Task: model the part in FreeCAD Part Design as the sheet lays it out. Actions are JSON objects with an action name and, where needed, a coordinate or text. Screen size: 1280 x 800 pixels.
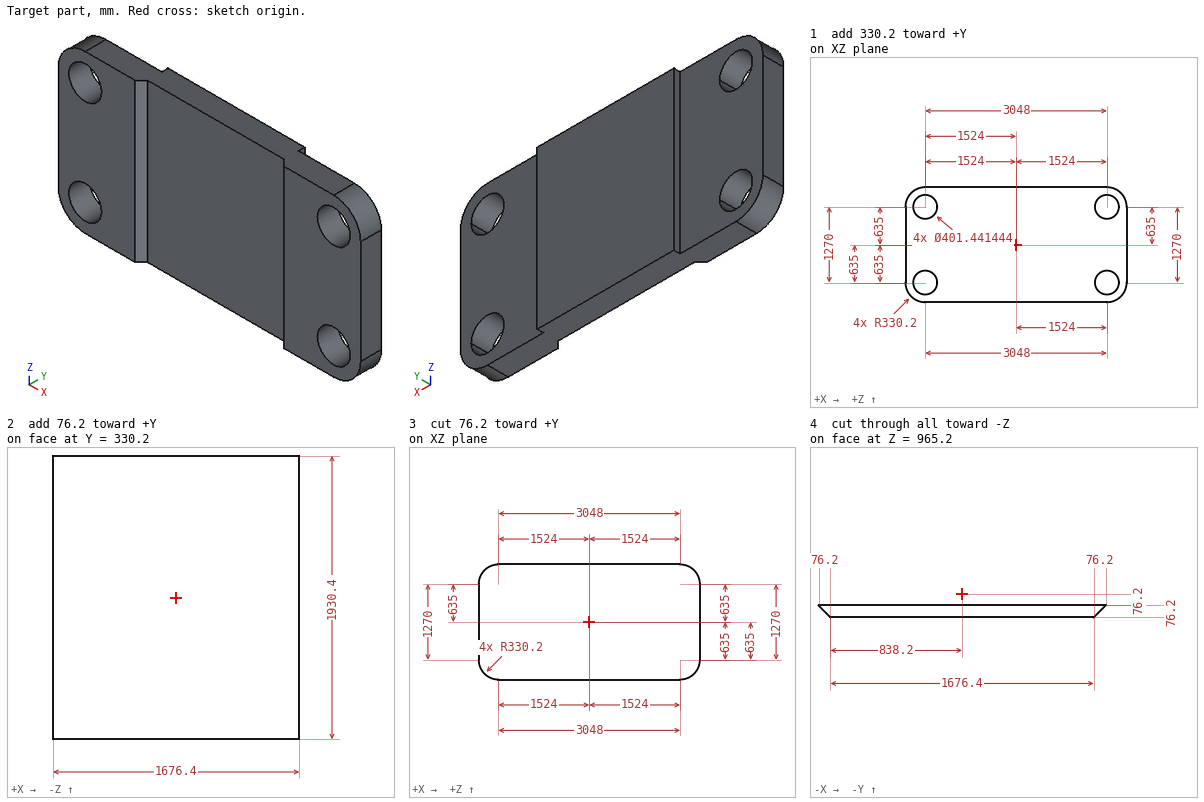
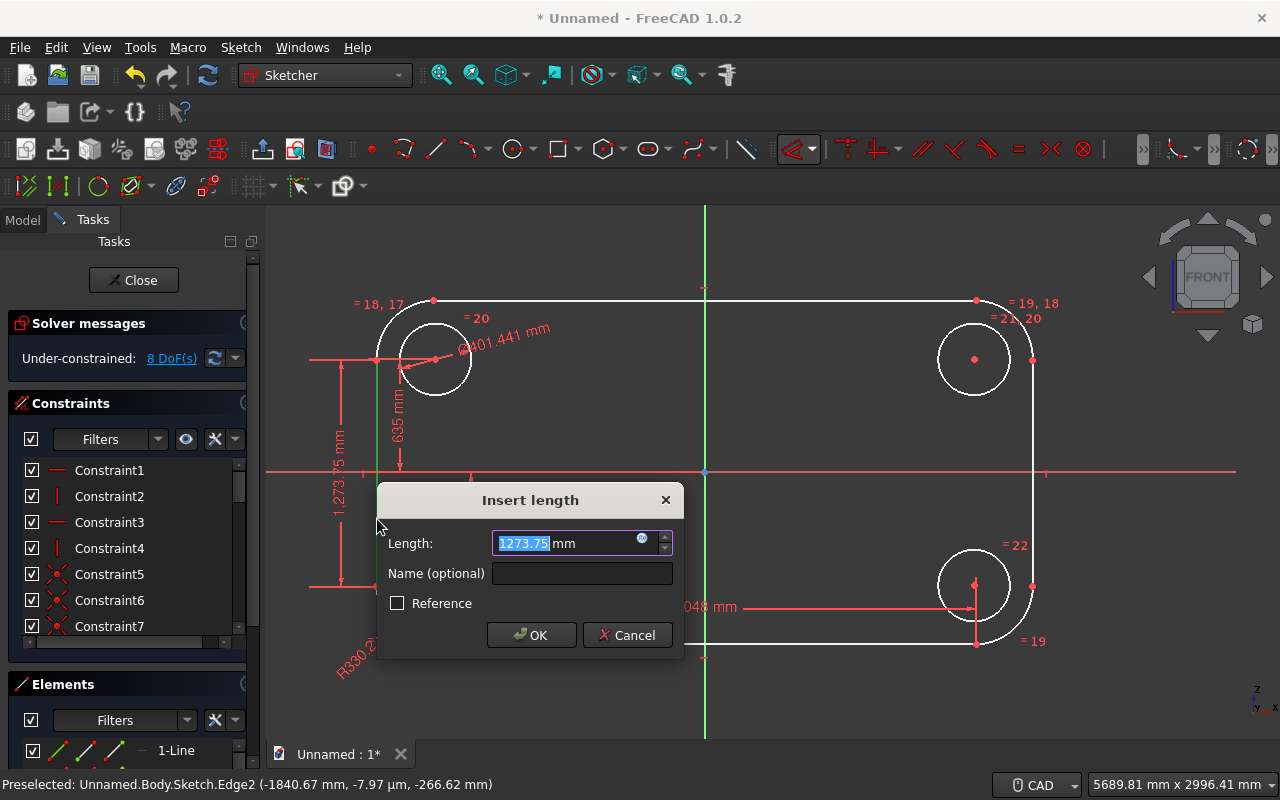
{"action": "type", "text": "1270"}
{"action": "key", "text": "Return"}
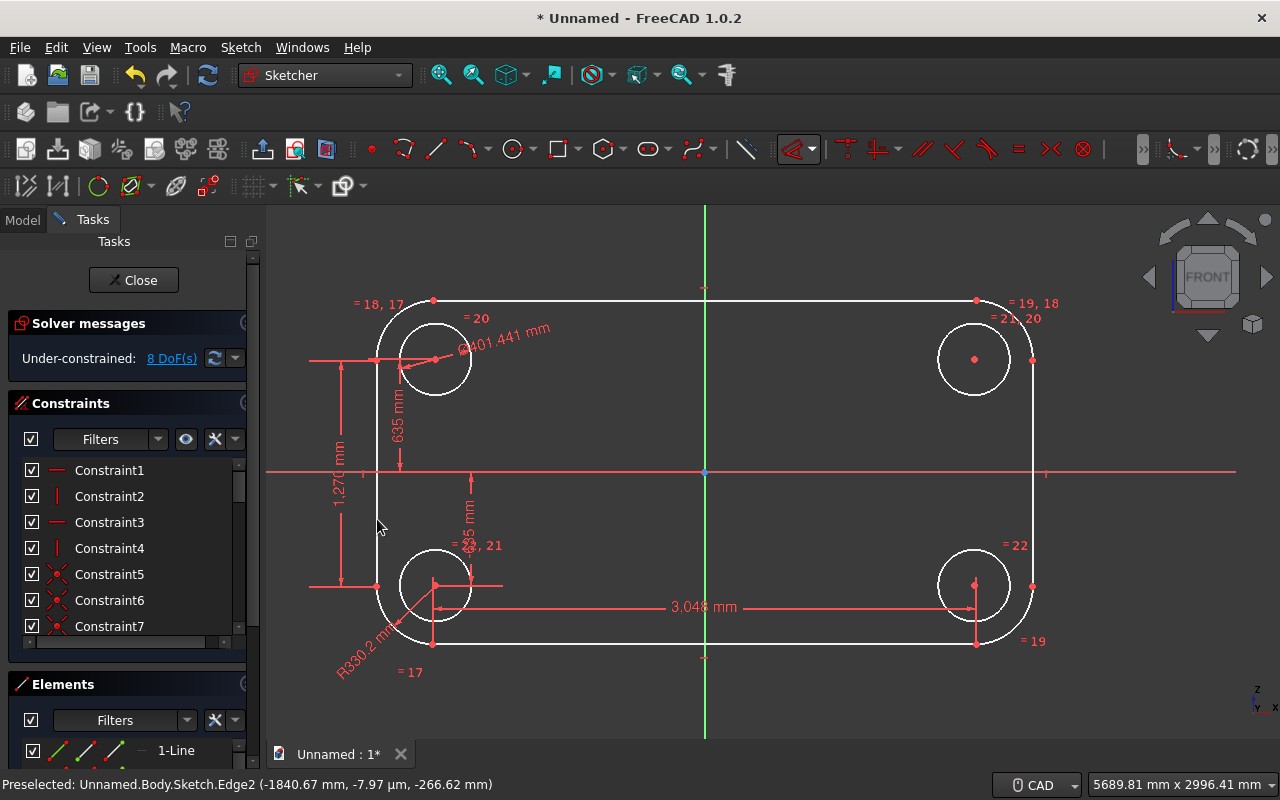
{"action": "left_click", "coordinate": [596, 301]}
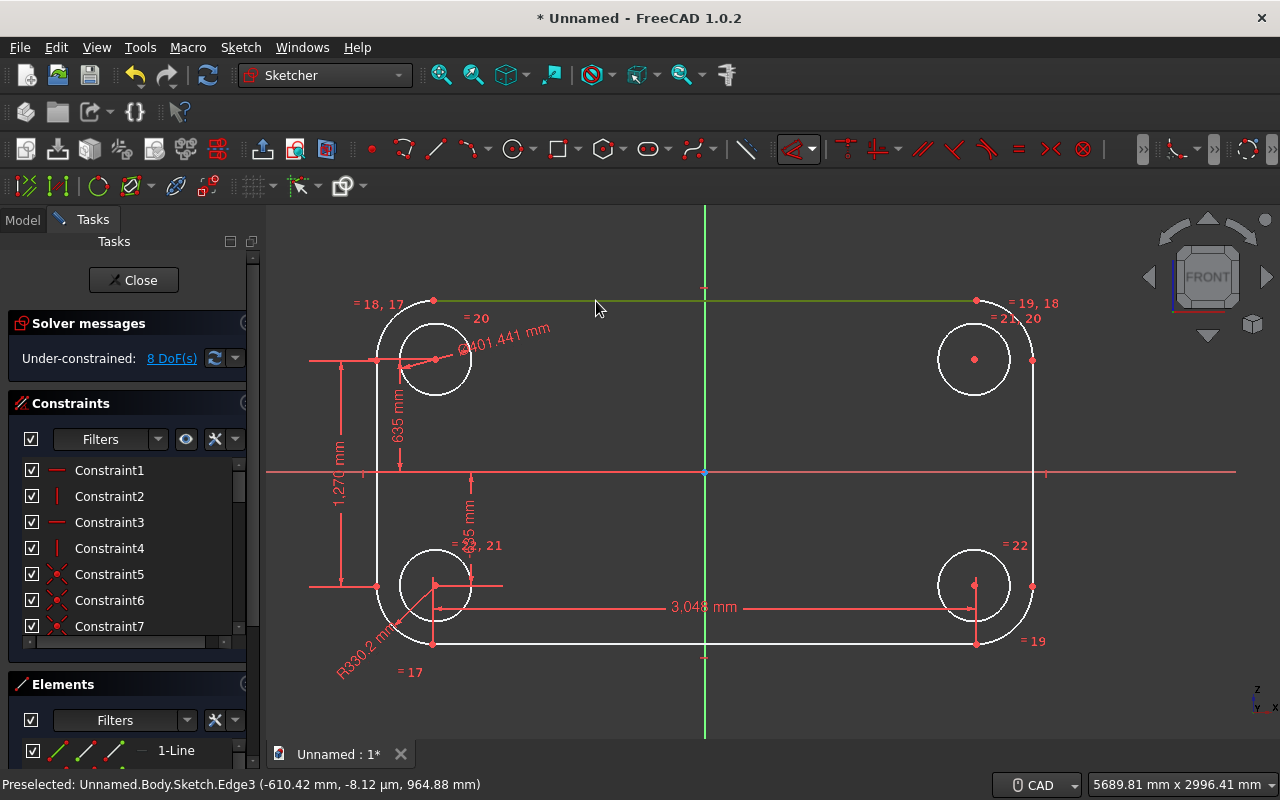
{"action": "left_click", "coordinate": [814, 150]}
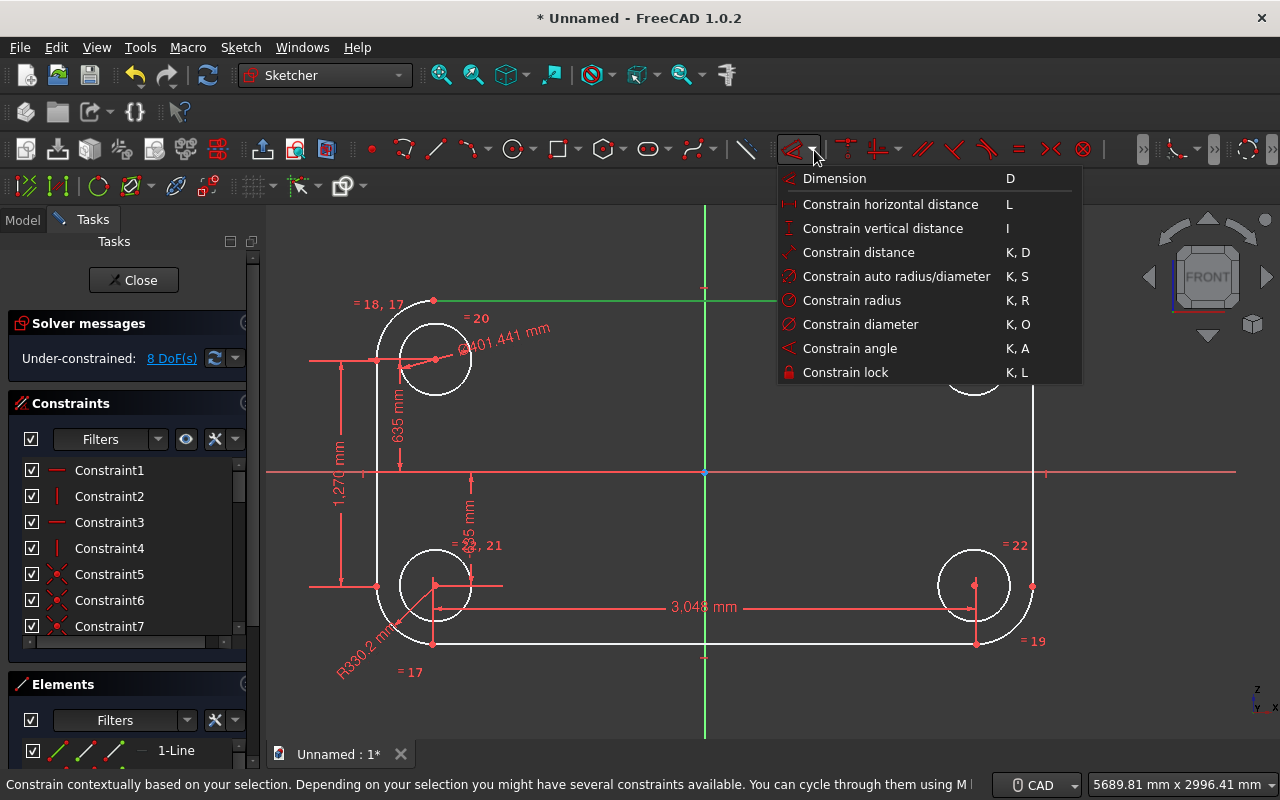
{"action": "left_click", "coordinate": [930, 204]}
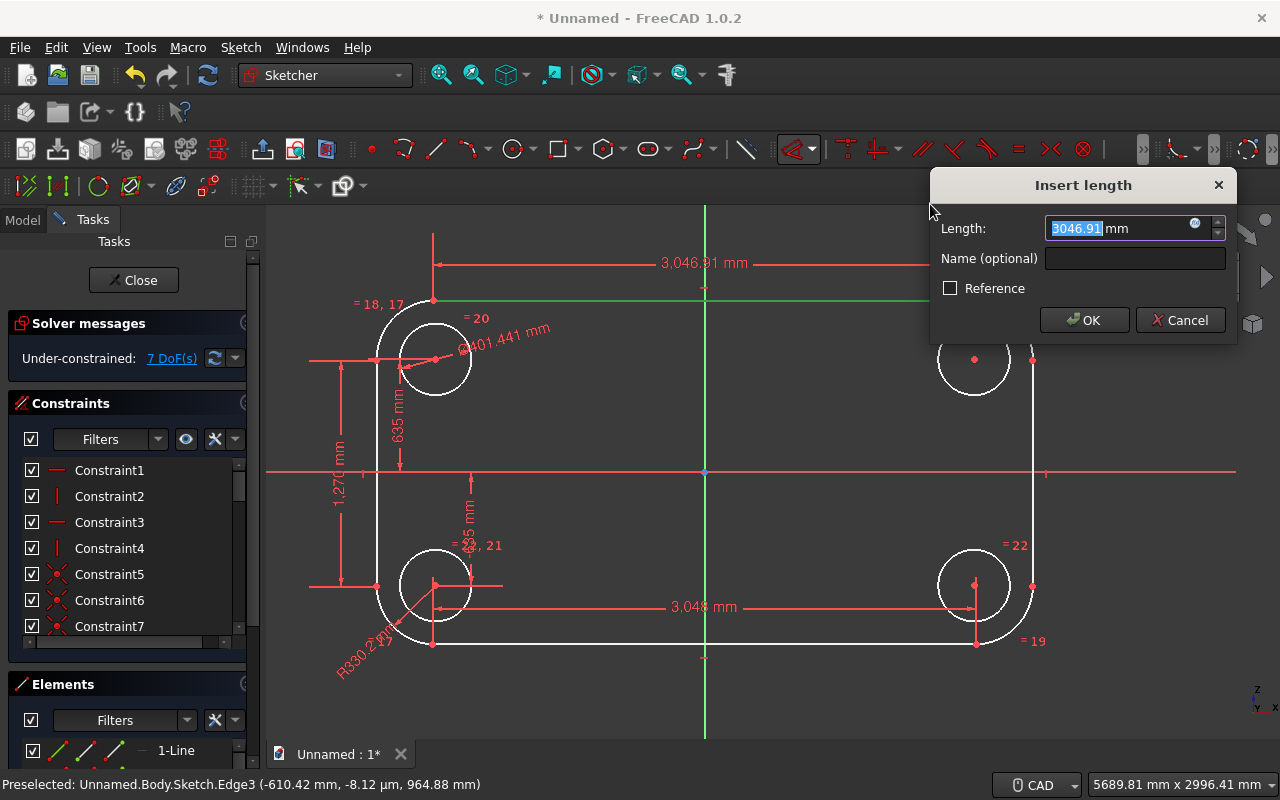
{"action": "type", "text": "3048"}
{"action": "key", "text": "Return"}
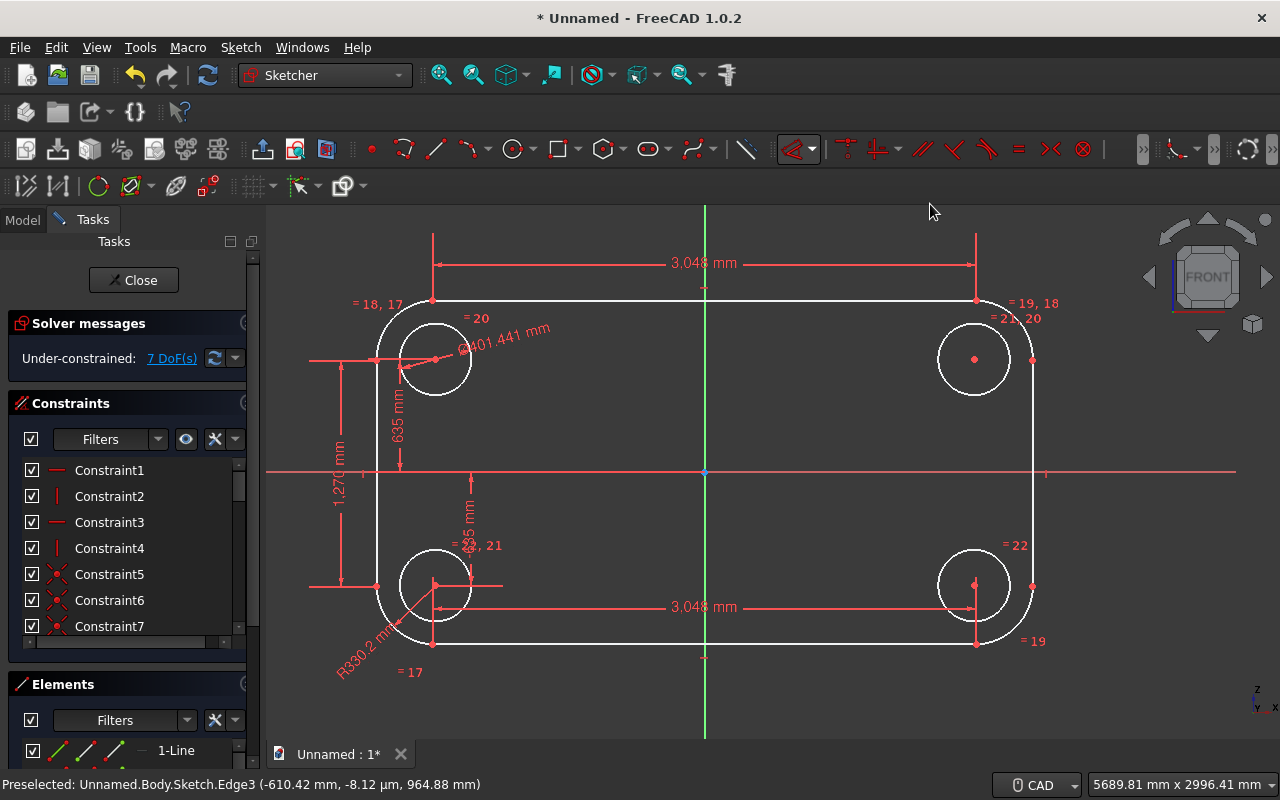
{"action": "left_click", "coordinate": [1033, 428]}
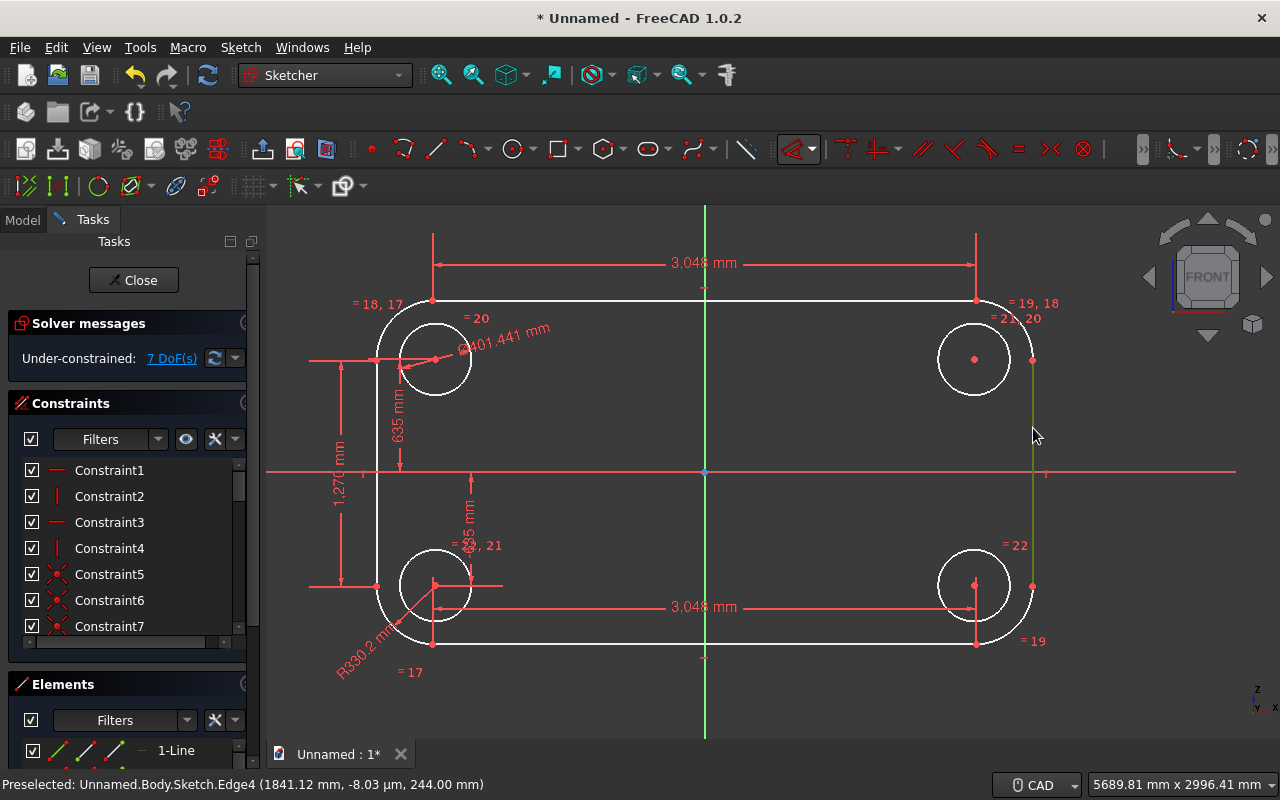
{"action": "key", "text": "i"}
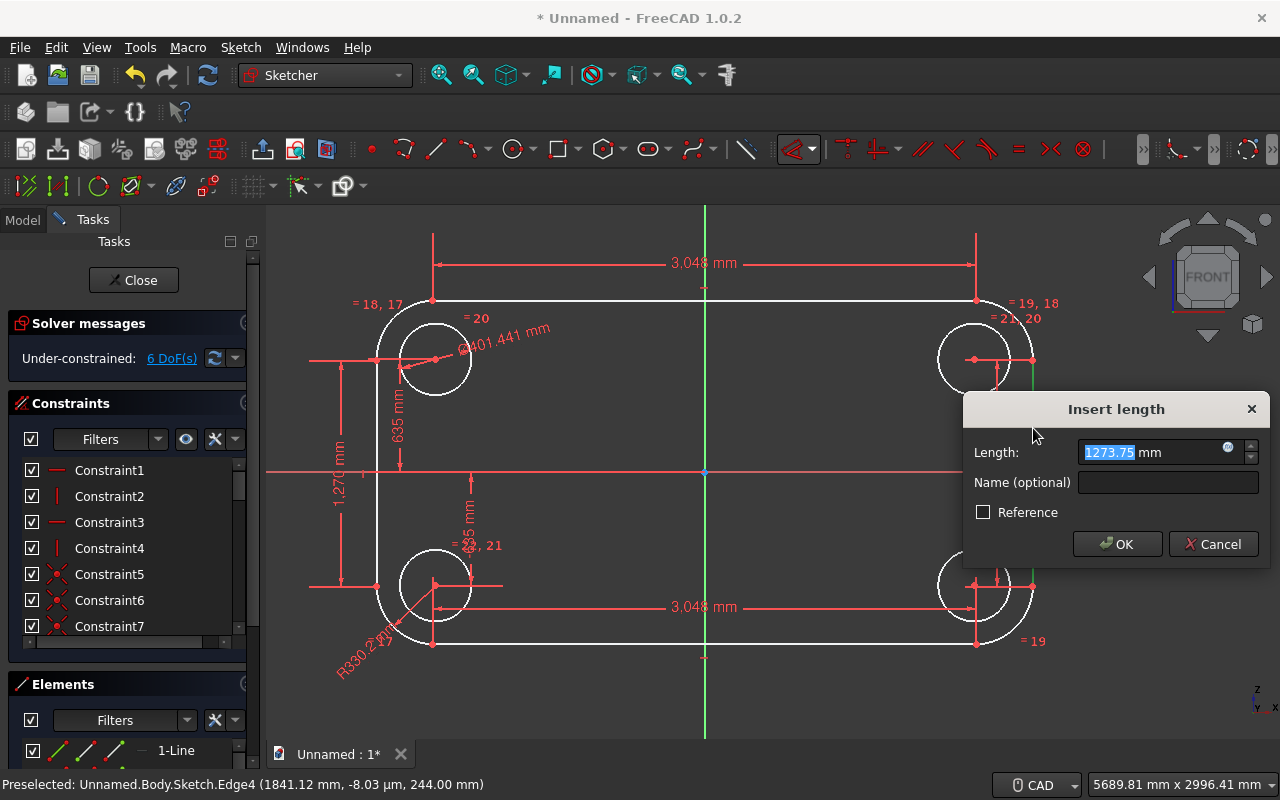
{"action": "type", "text": "1270"}
{"action": "key", "text": "Return"}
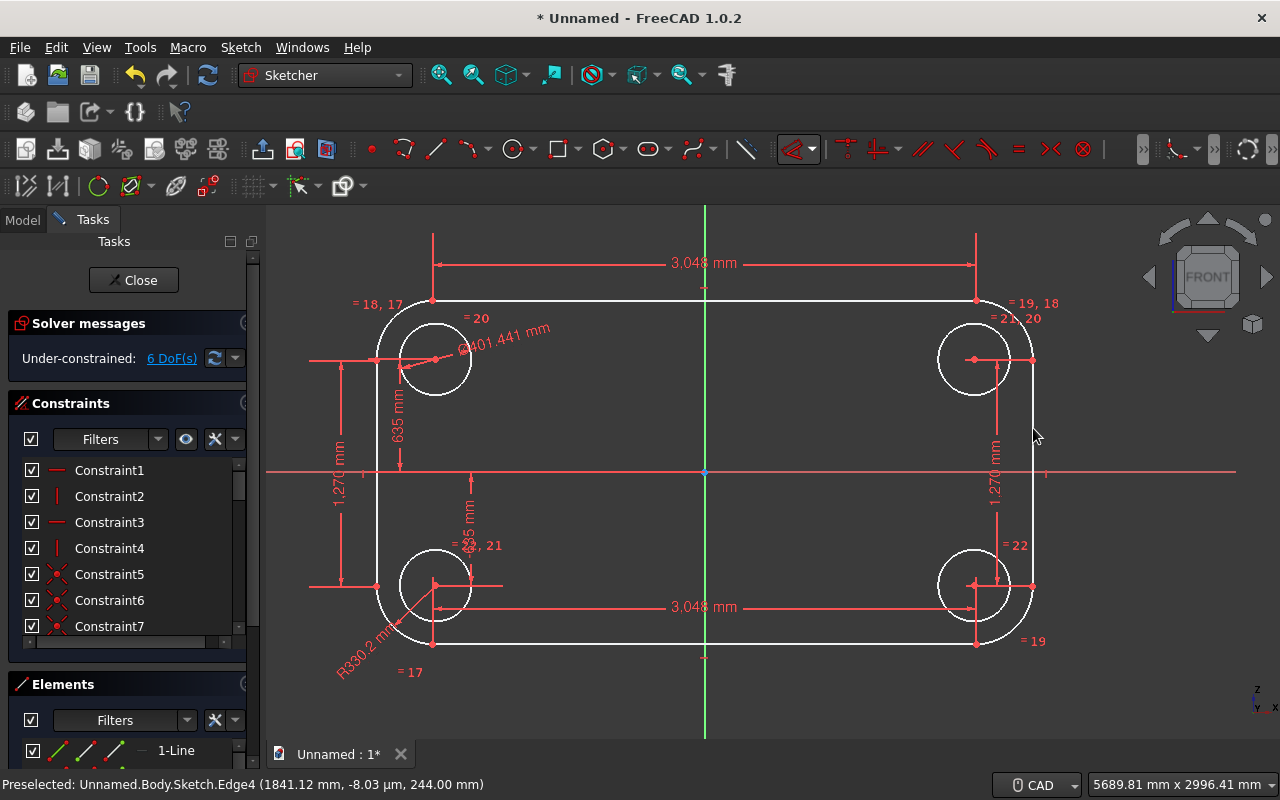
{"action": "left_click", "coordinate": [377, 587]}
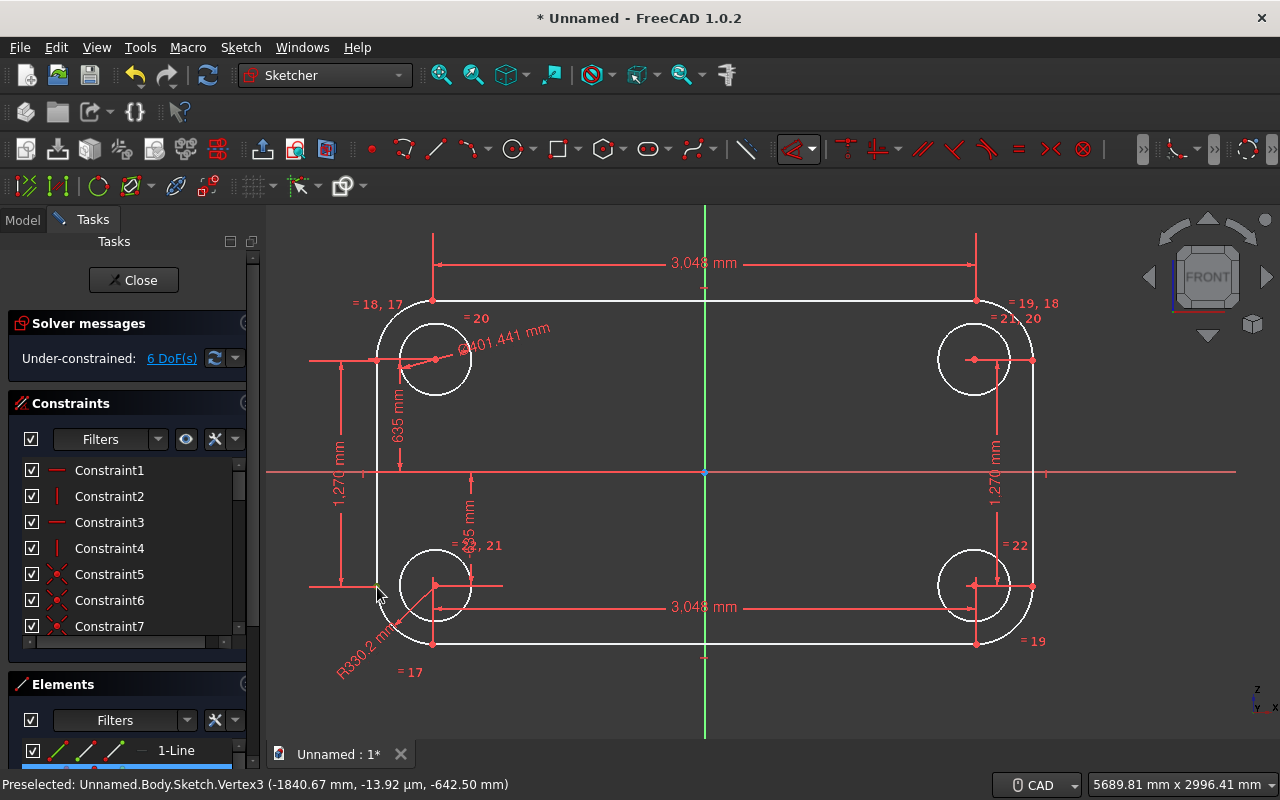
{"action": "key", "text": "i"}